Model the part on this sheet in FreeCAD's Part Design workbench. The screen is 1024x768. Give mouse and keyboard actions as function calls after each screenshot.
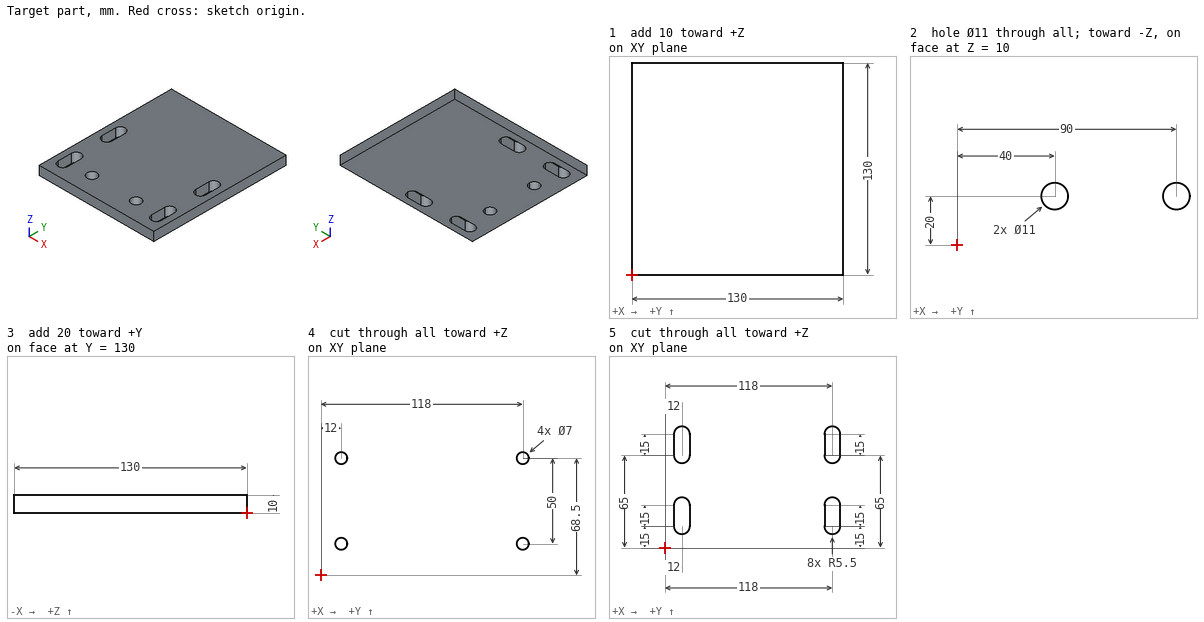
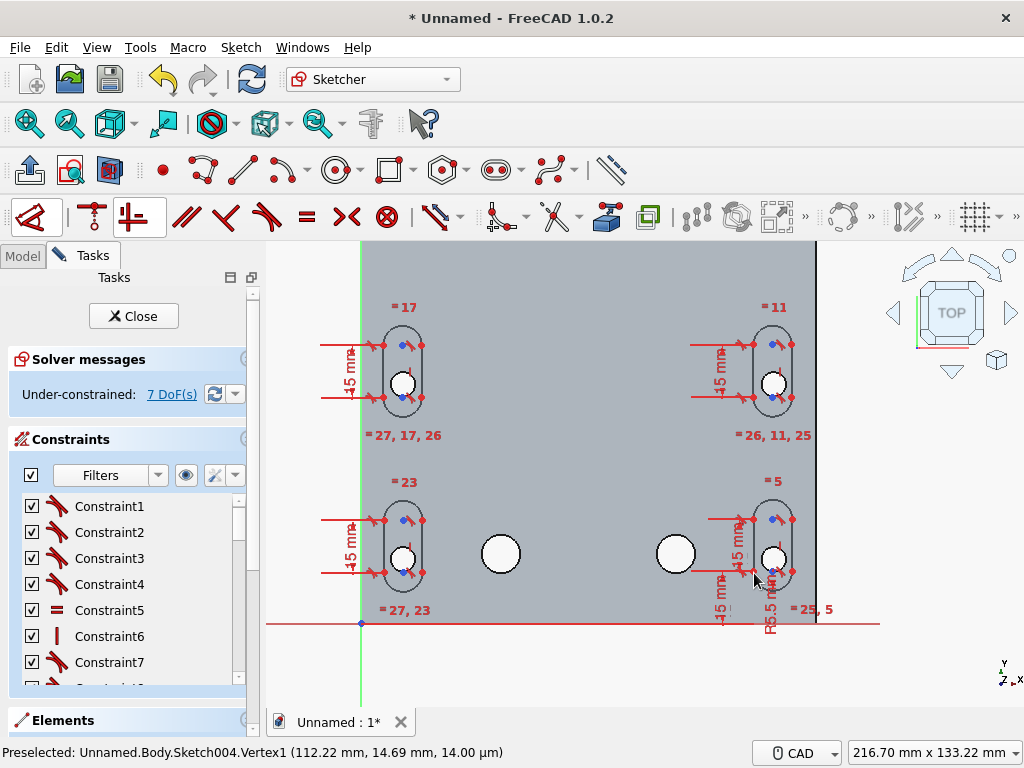
click(754, 397)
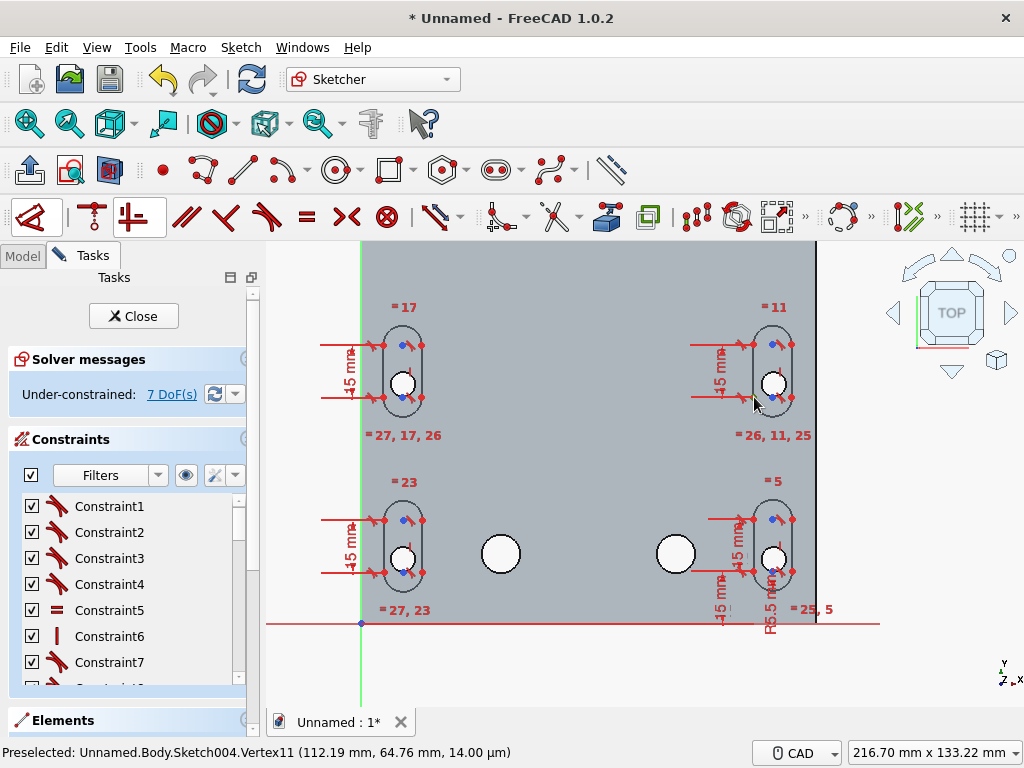
key(i)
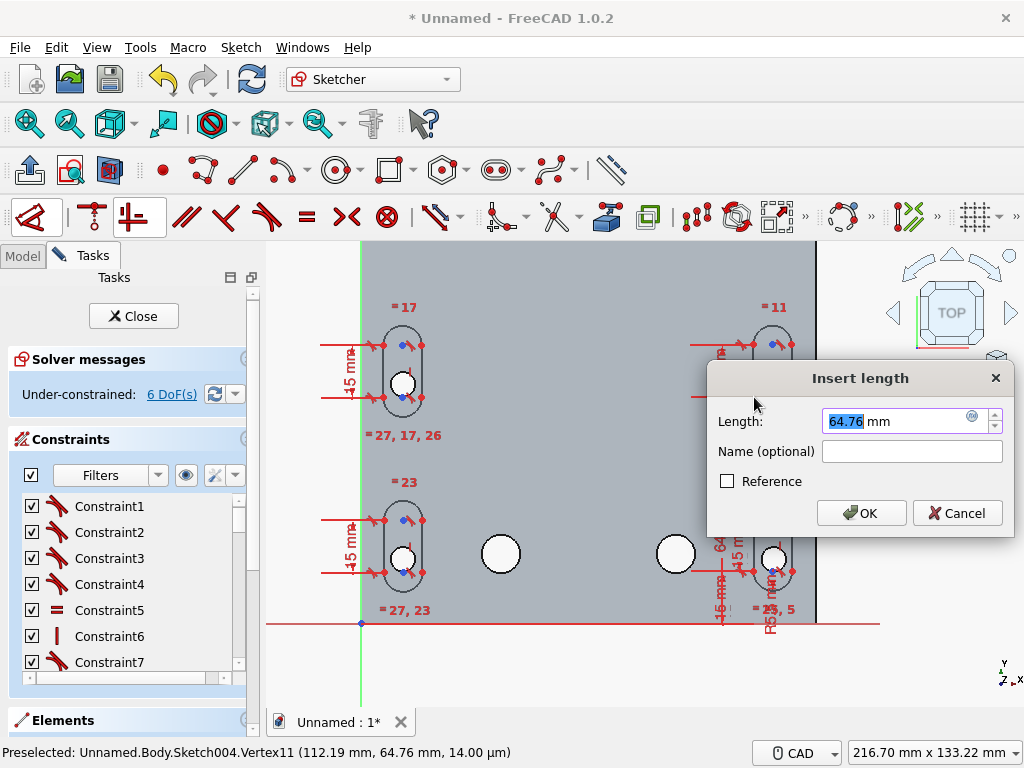
text(65)
key(Return)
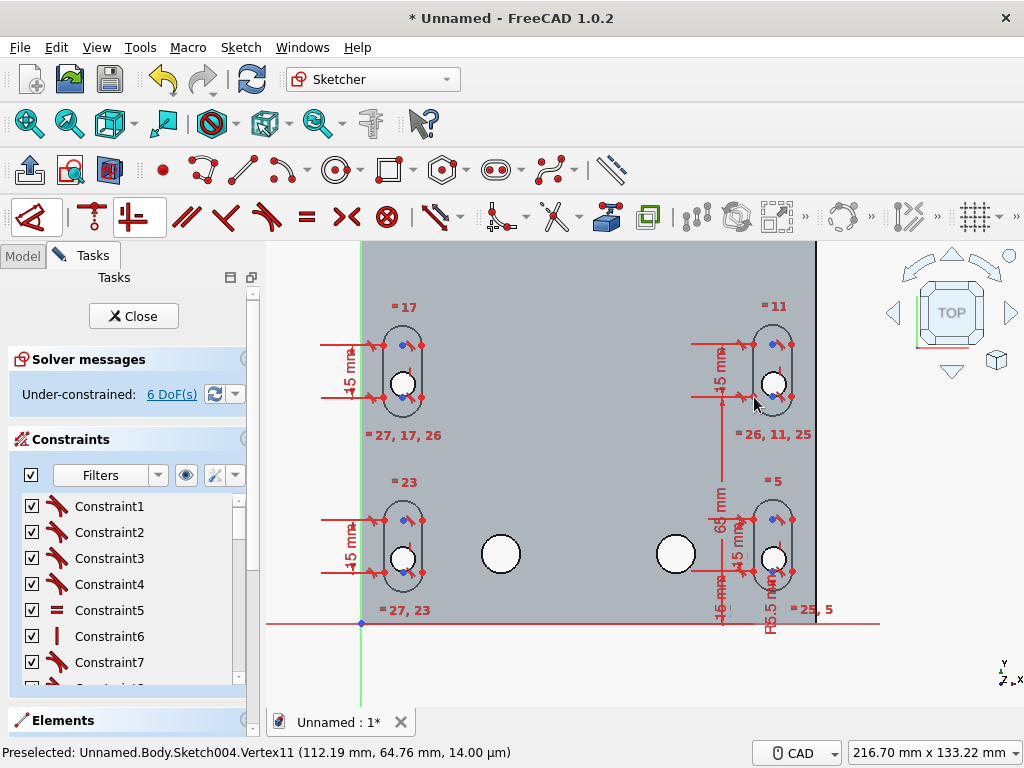
click(383, 398)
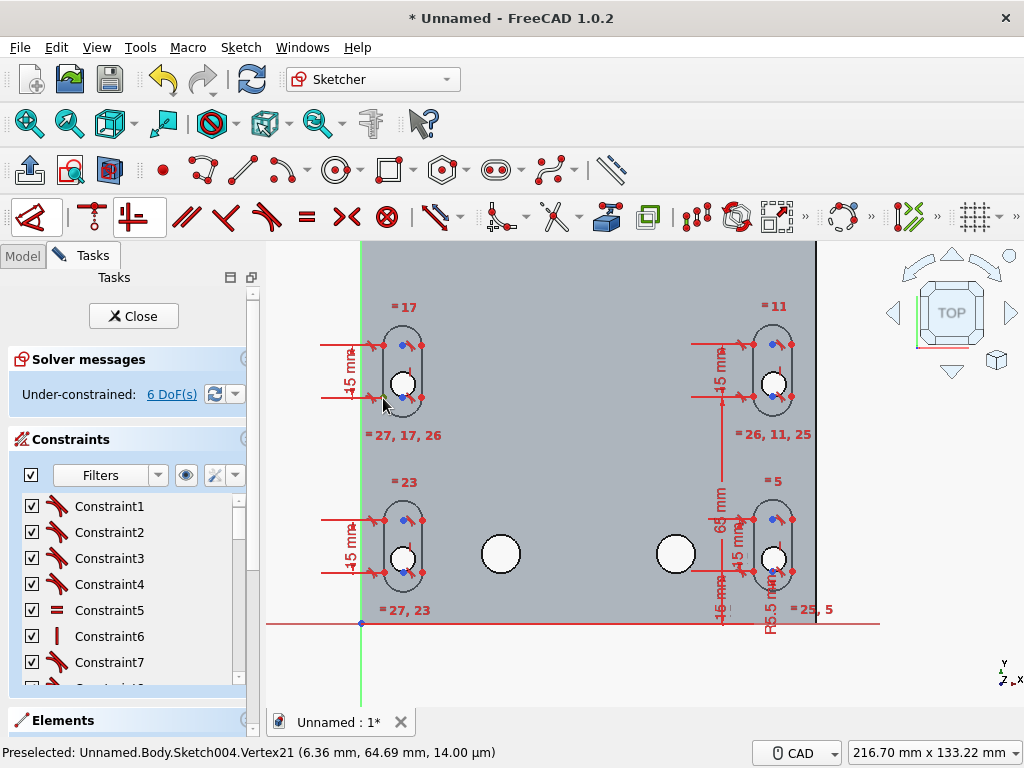
key(i)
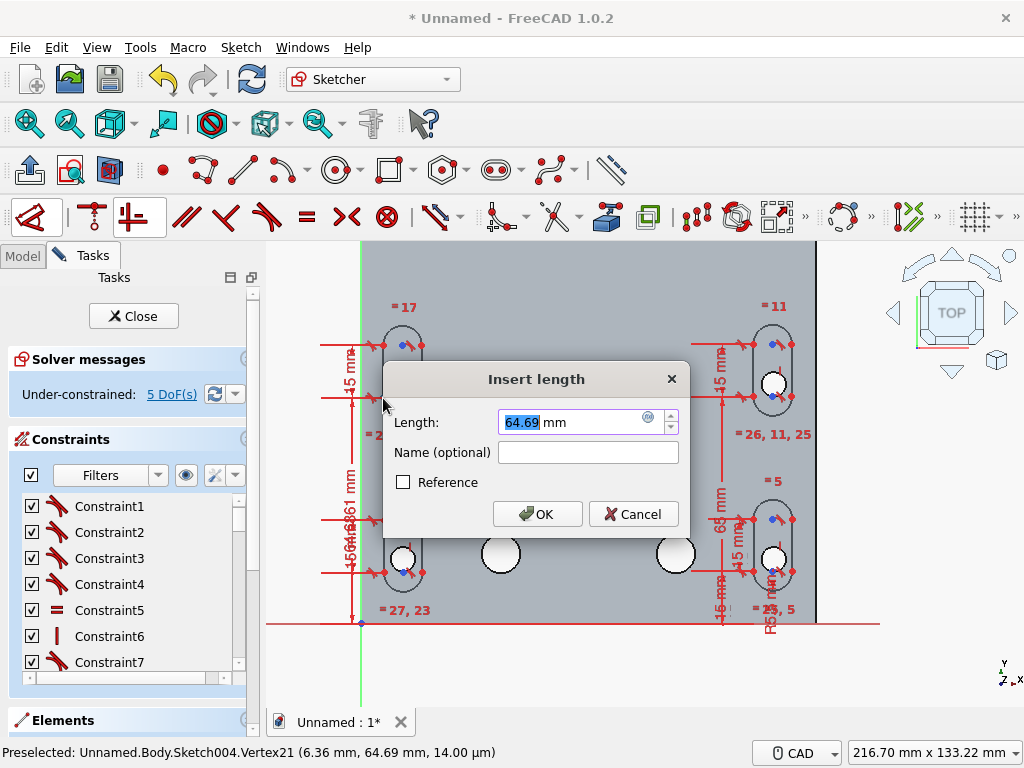
text(65)
key(Return)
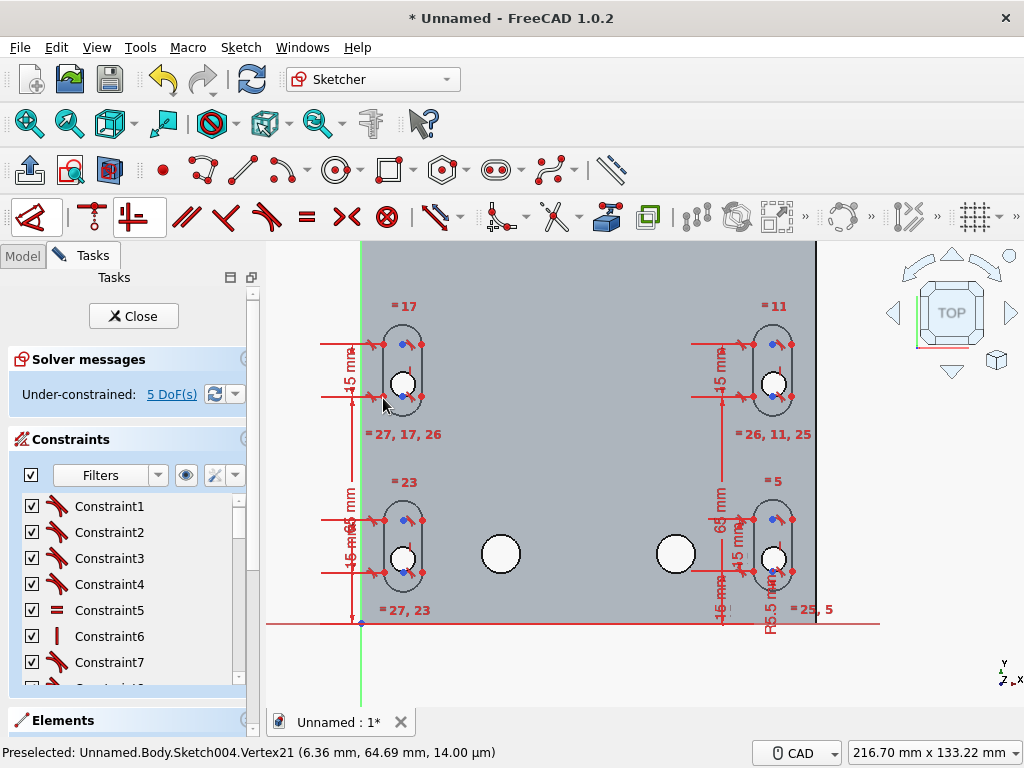
click(384, 573)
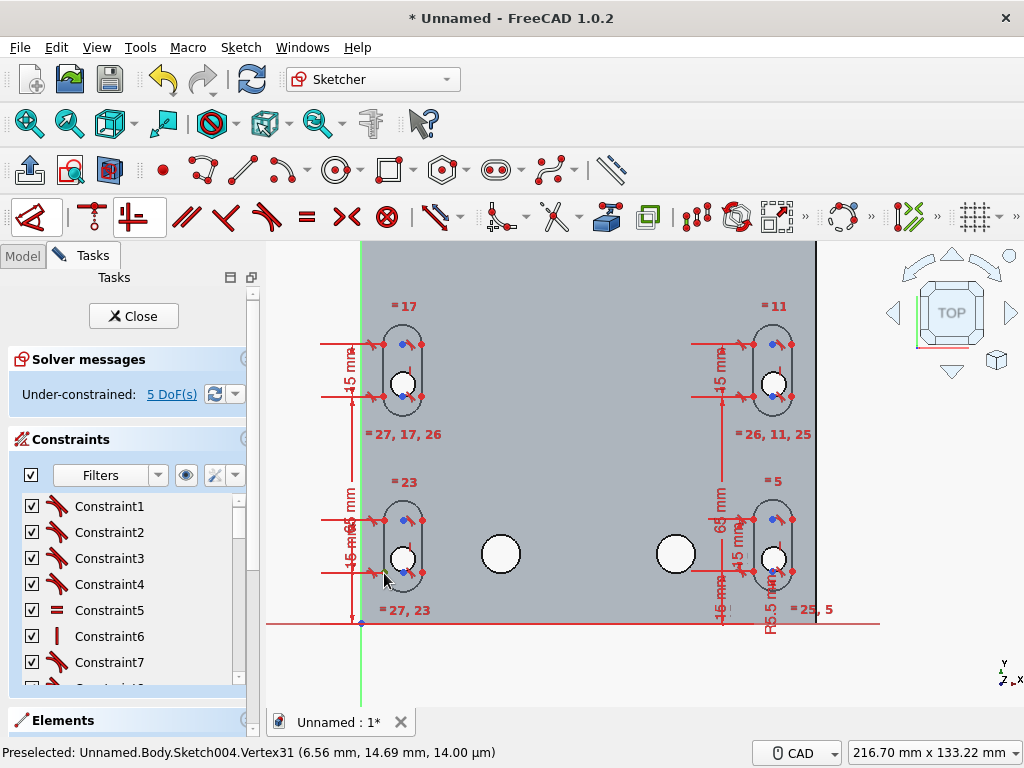
key(i)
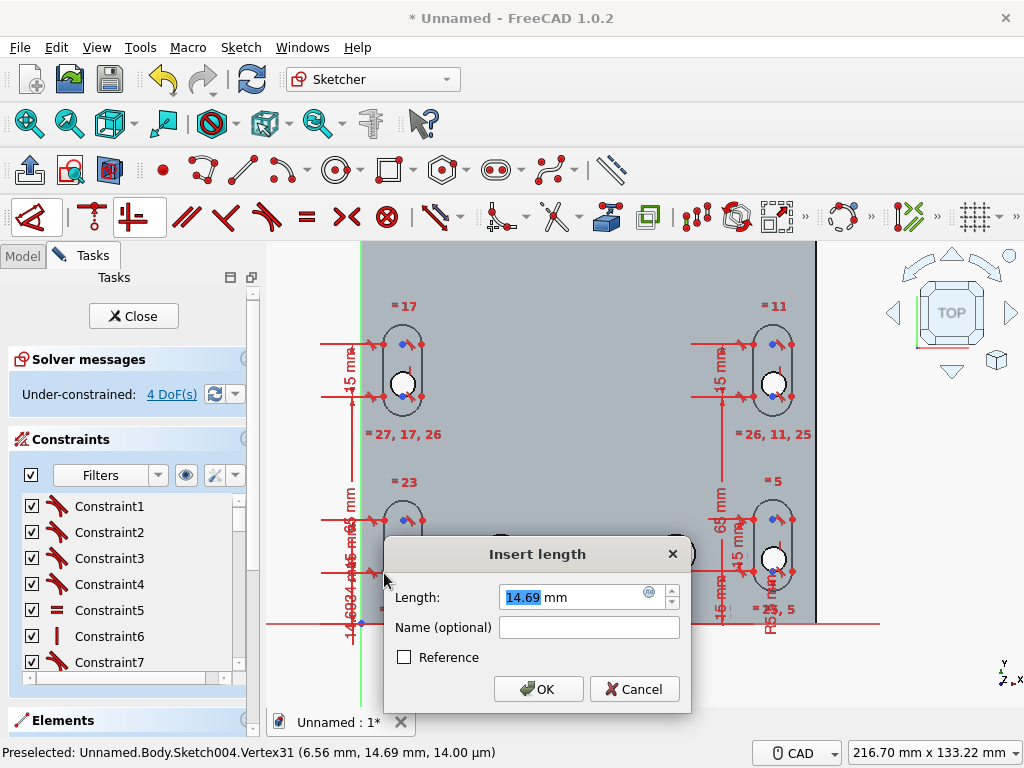
text(15)
key(Return)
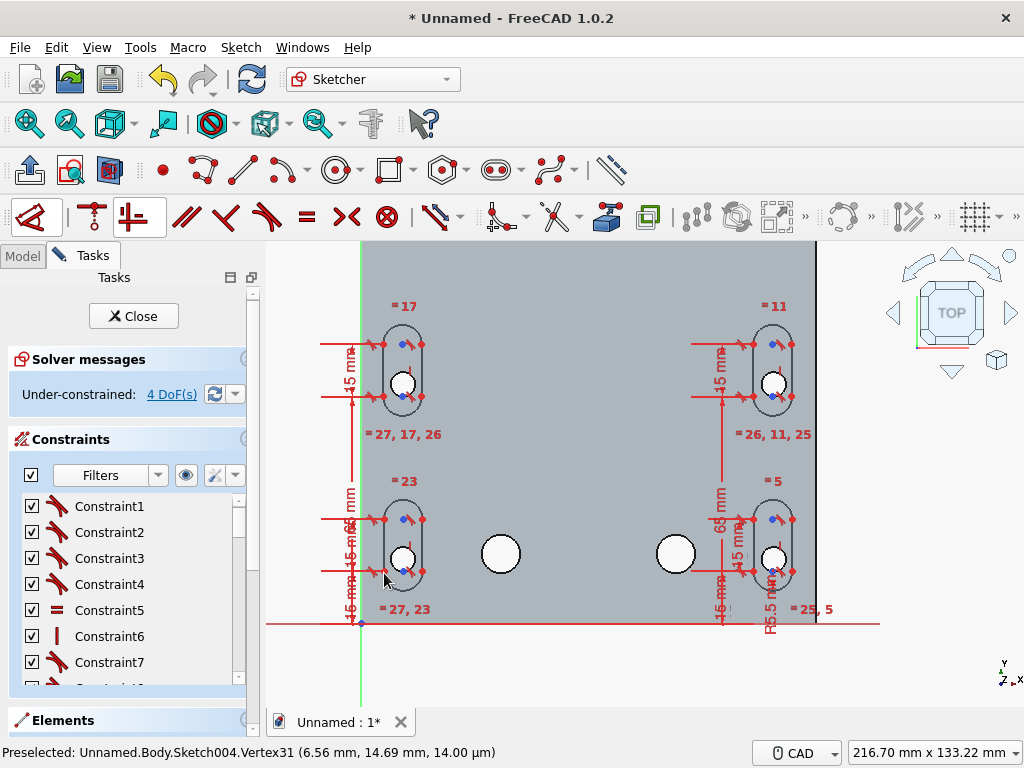
click(403, 397)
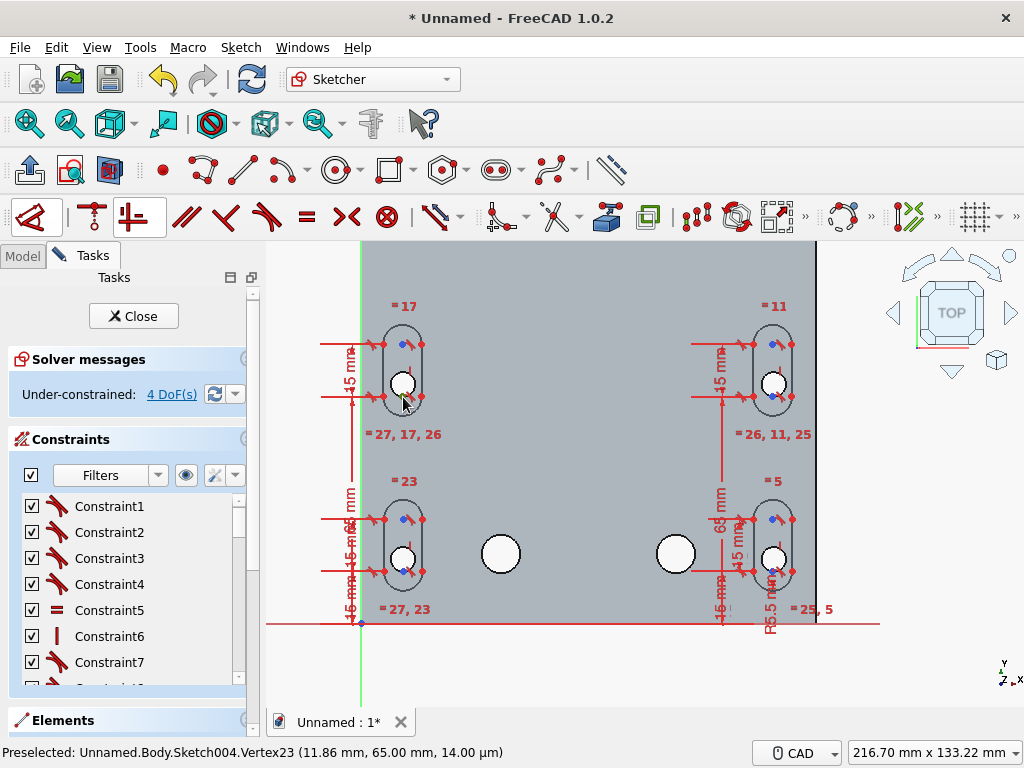
key(l)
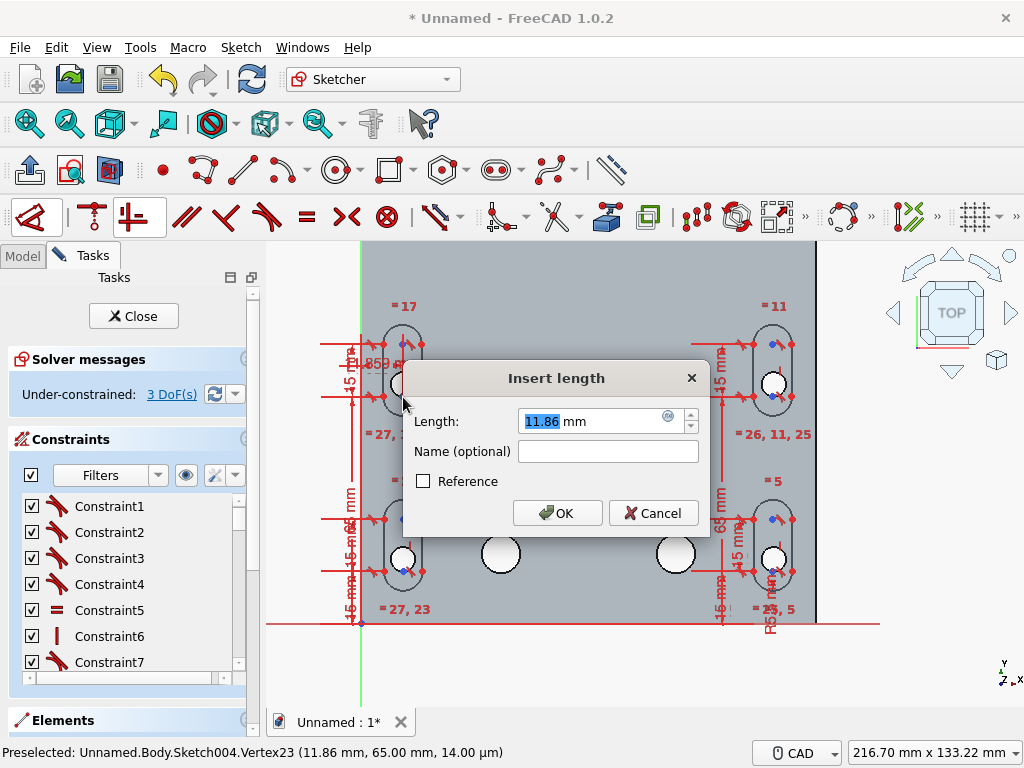
text(12)
key(Return)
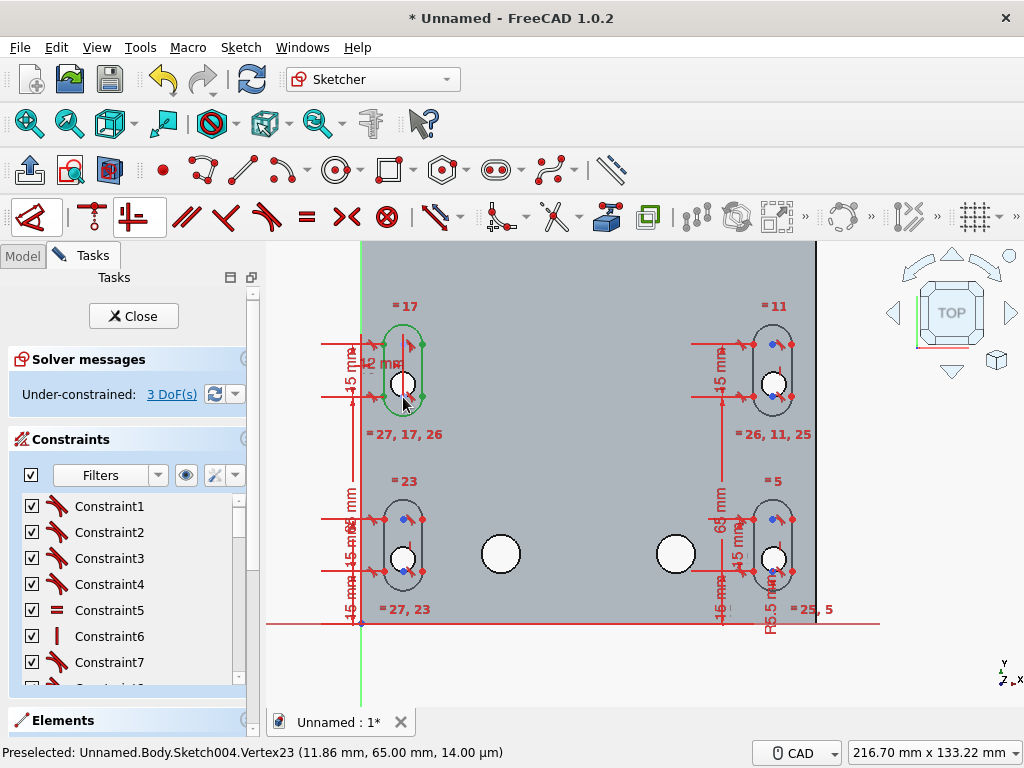
click(403, 571)